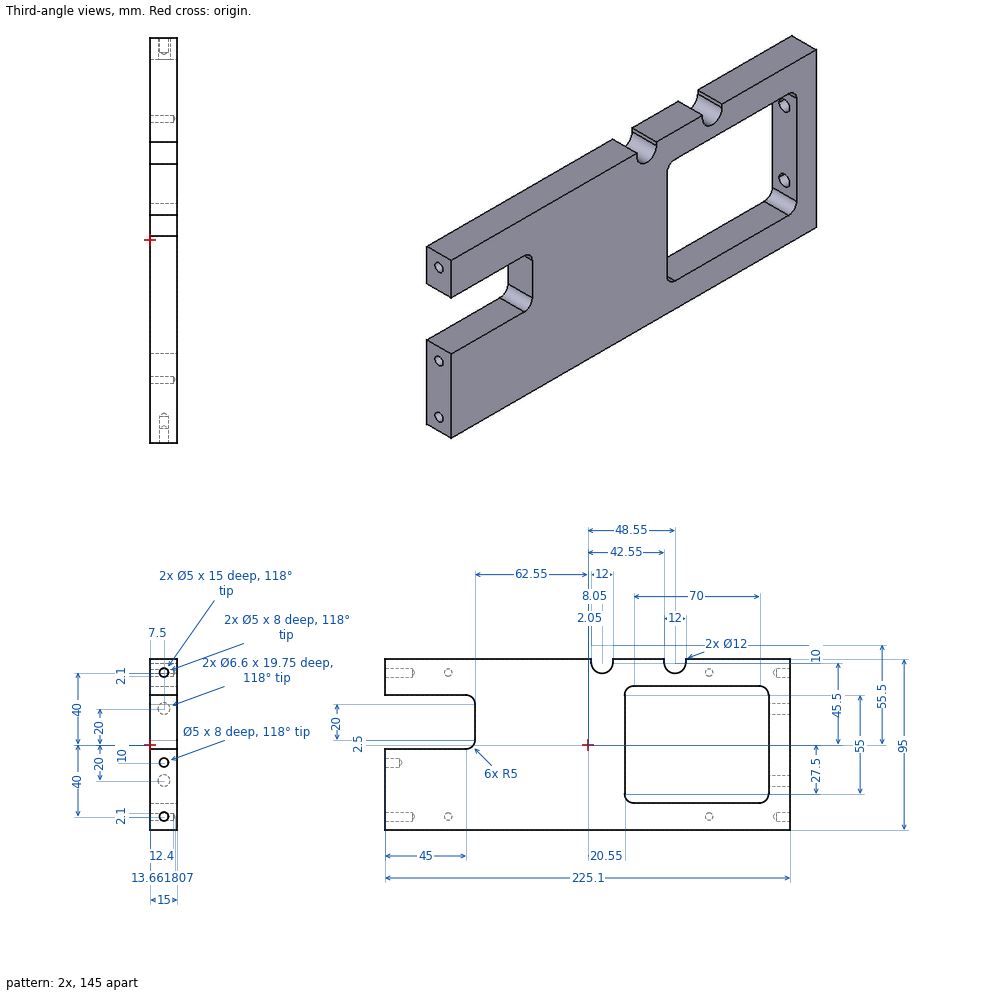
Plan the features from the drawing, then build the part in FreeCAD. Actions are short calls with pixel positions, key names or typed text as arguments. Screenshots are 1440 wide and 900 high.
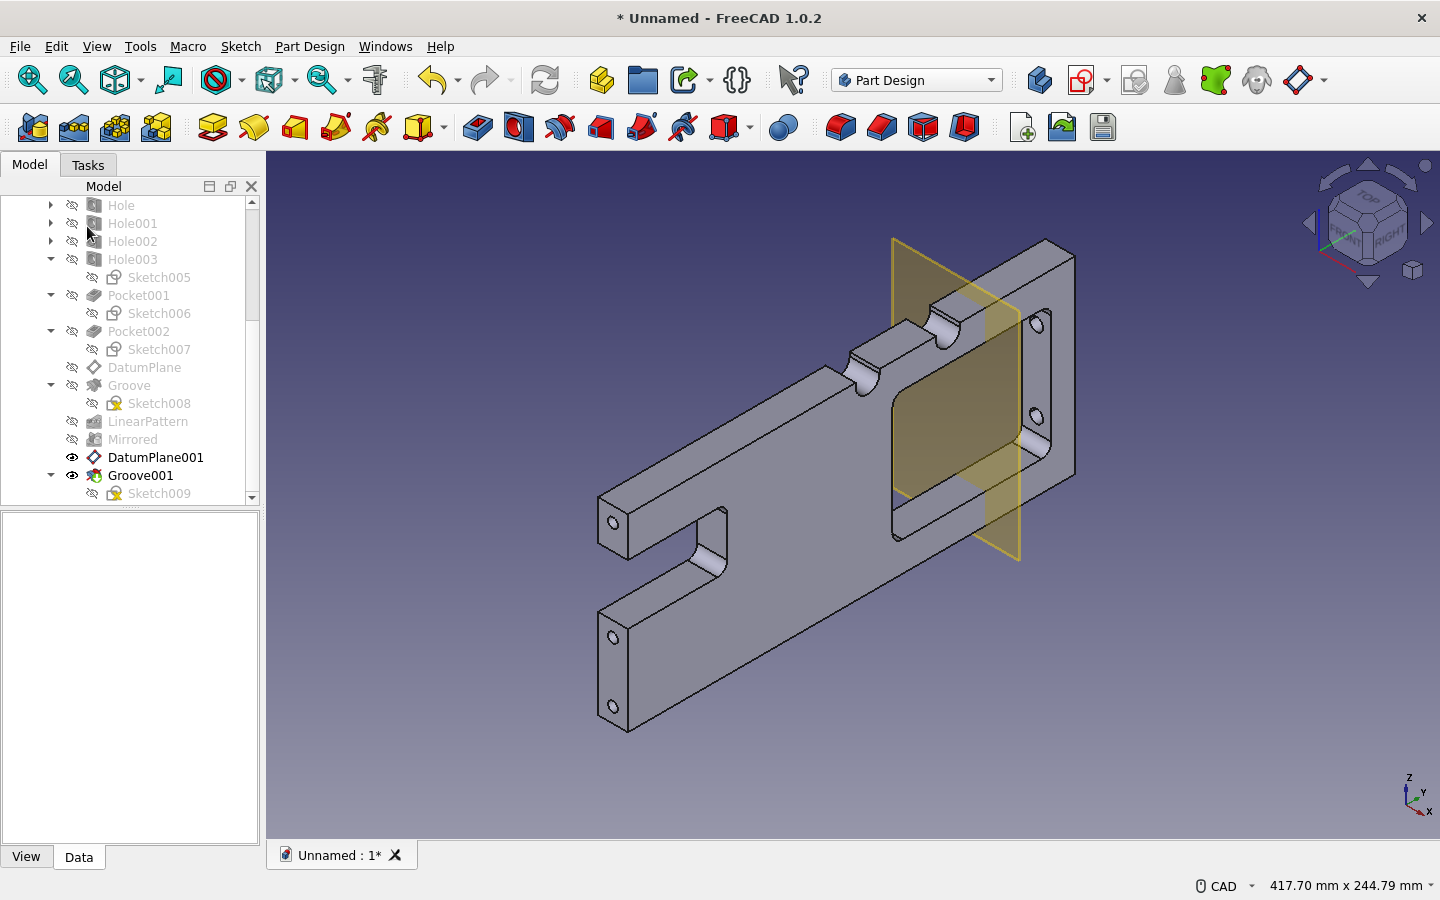
click(117, 457)
key(space)